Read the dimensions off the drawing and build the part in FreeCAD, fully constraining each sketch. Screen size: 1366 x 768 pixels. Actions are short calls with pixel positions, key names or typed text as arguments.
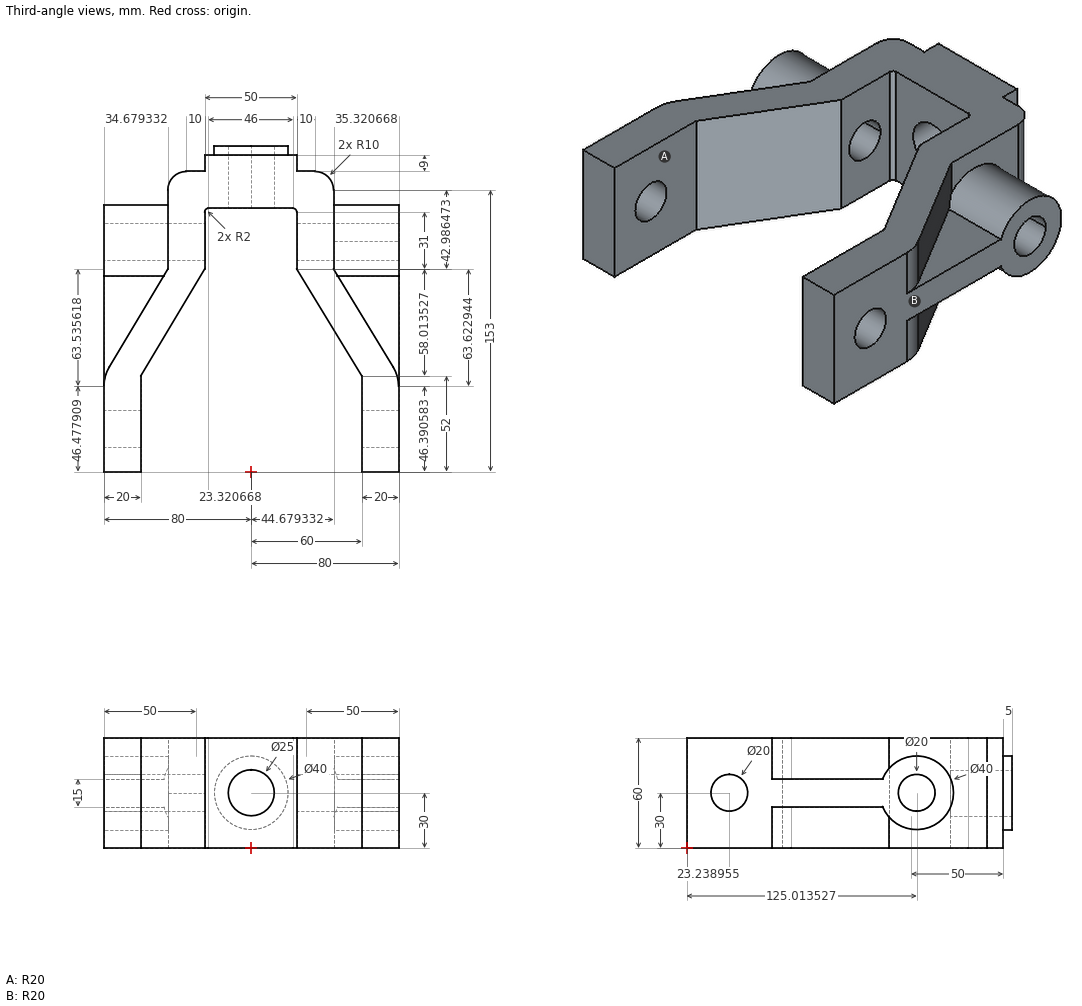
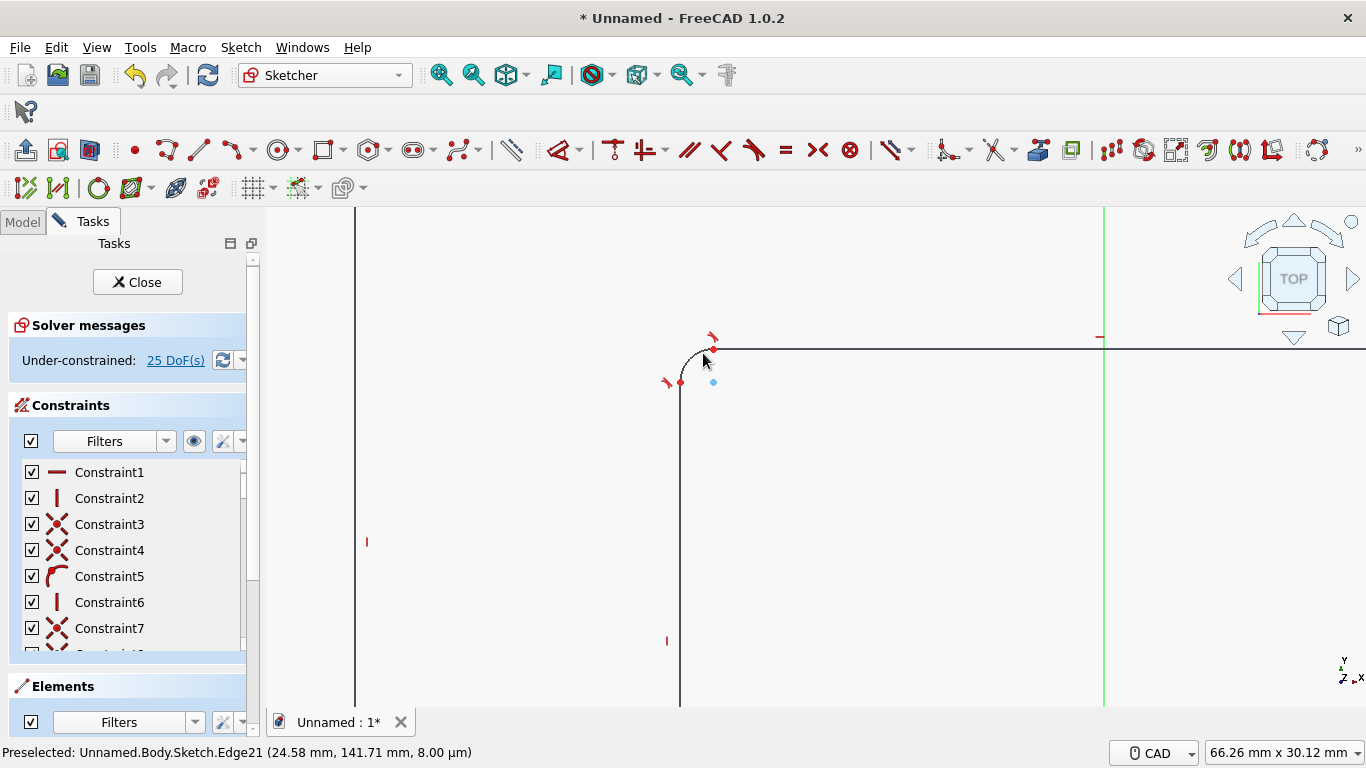
click(699, 353)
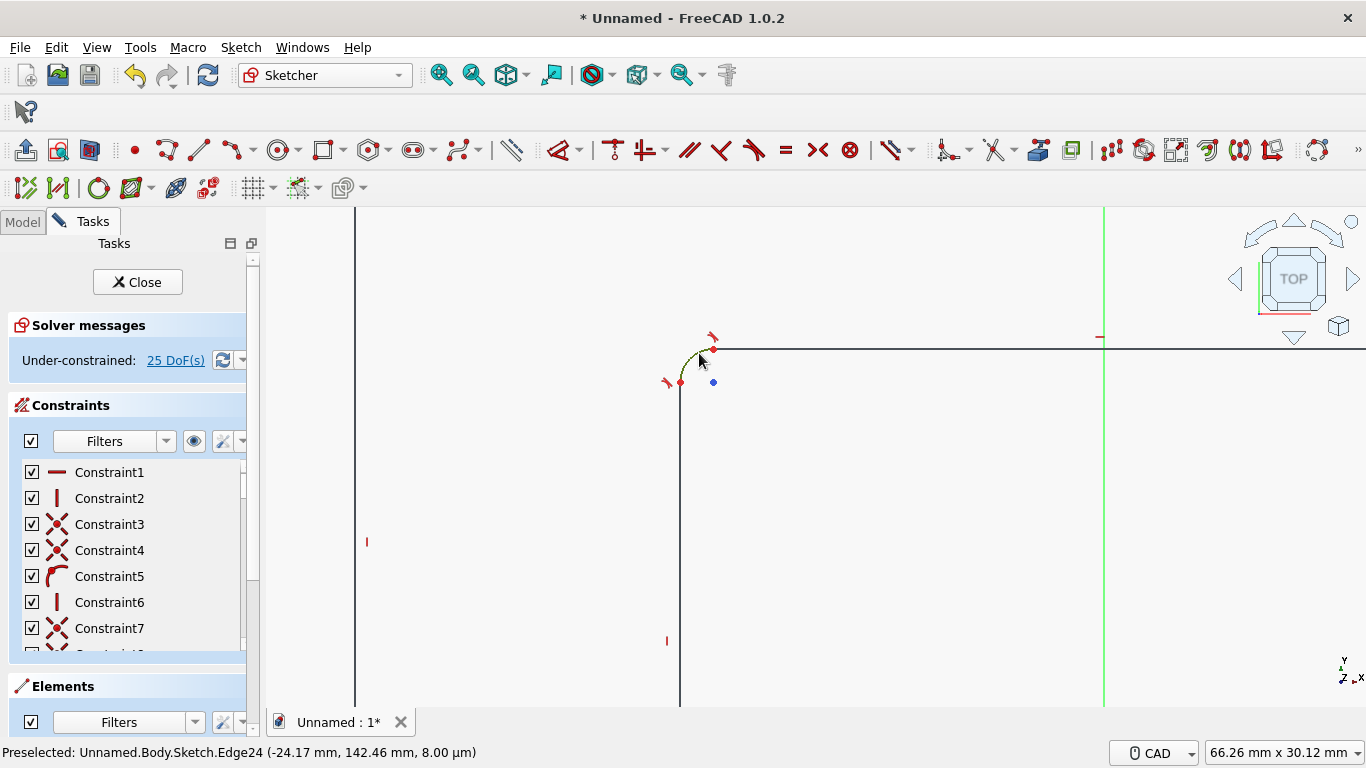
click(786, 150)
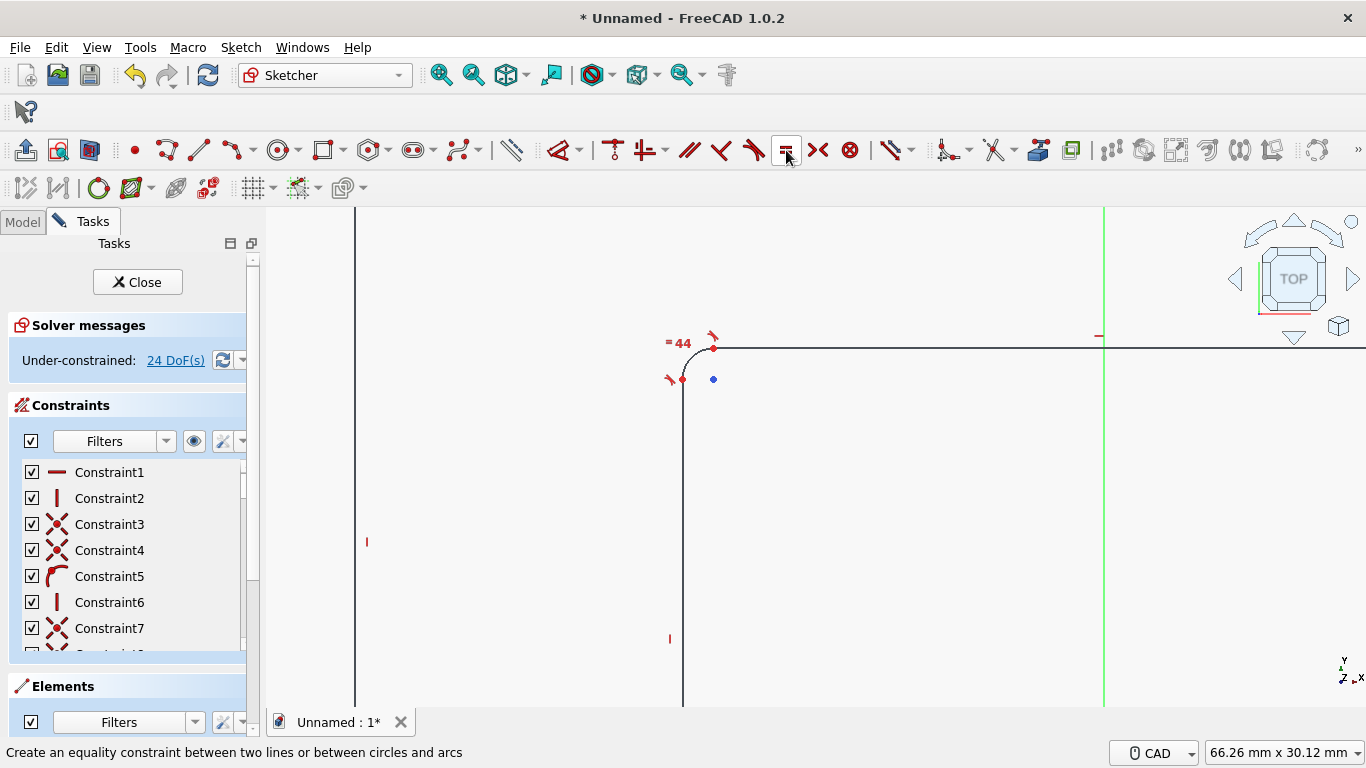
scroll(703, 353, down, 11)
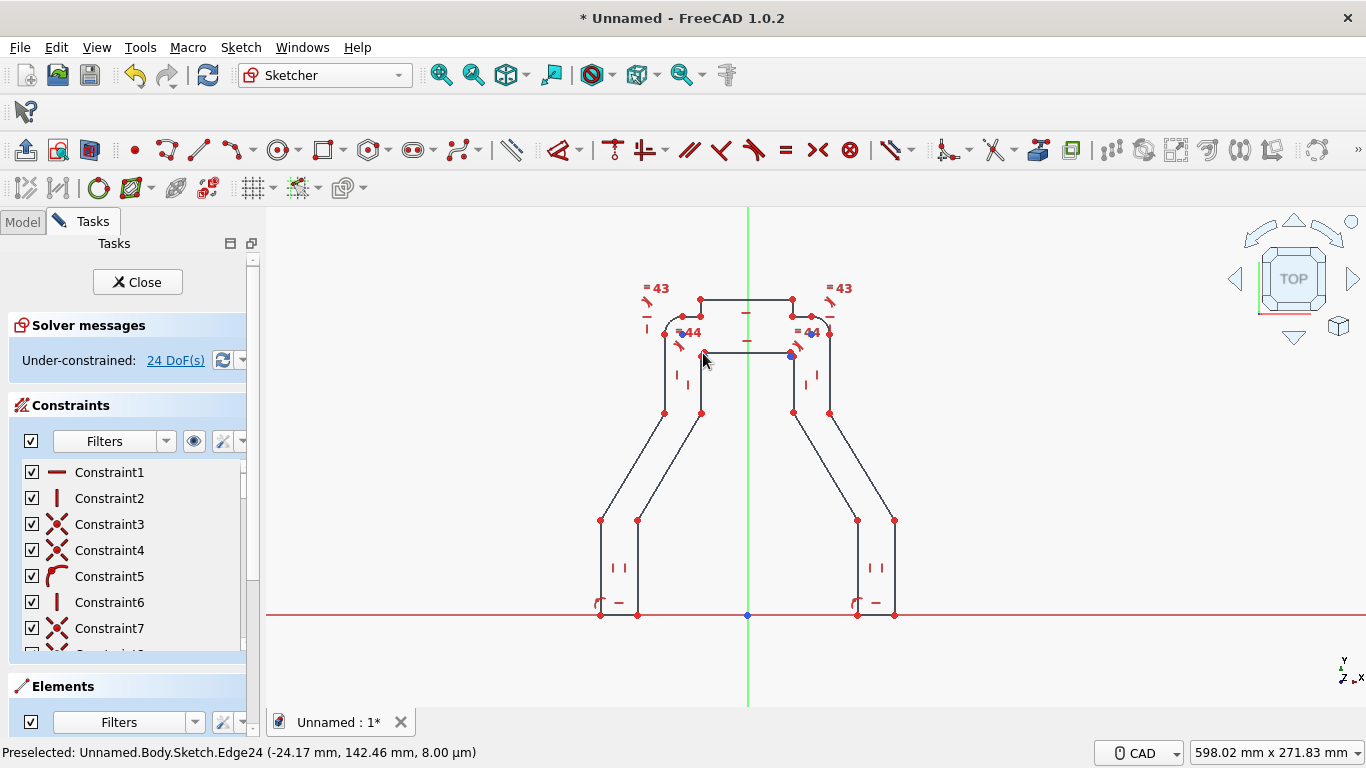
scroll(793, 355, up, 12)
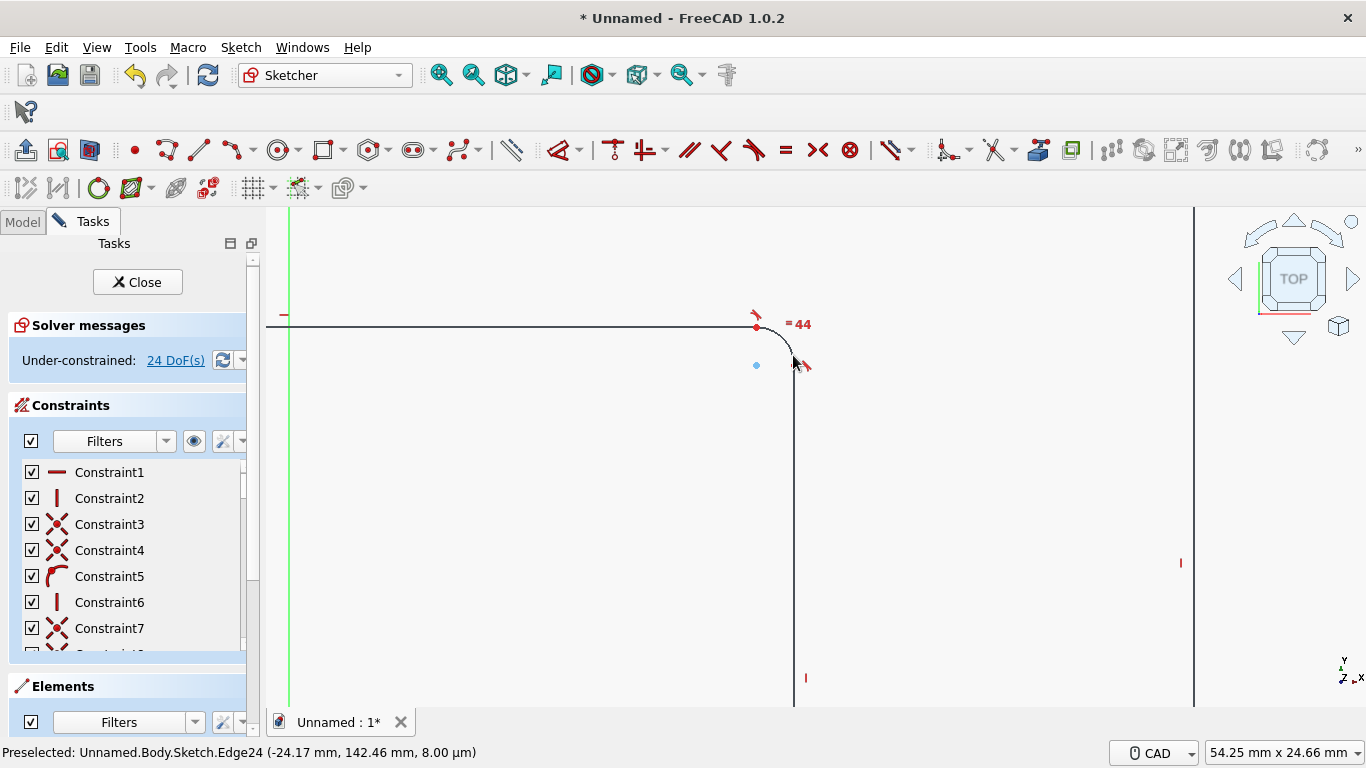
click(790, 348)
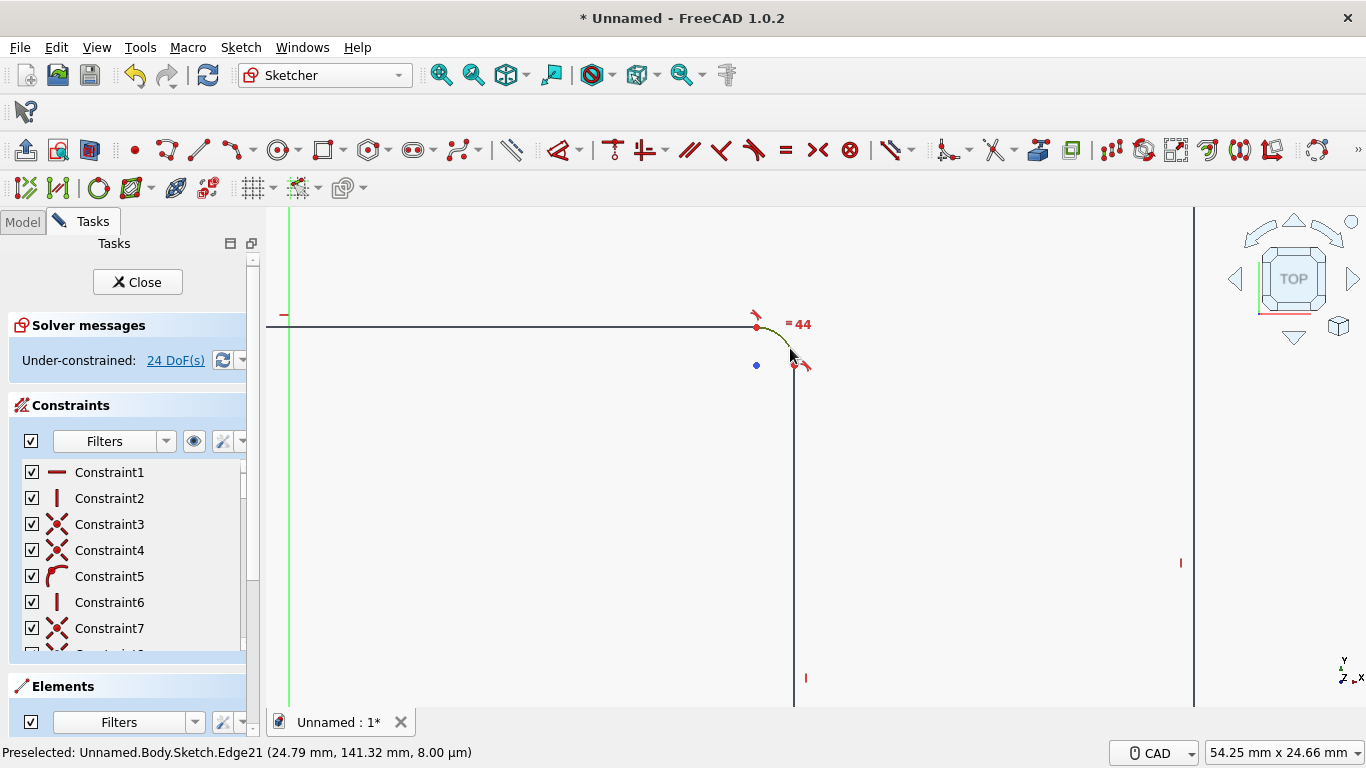
key(k)
key(r)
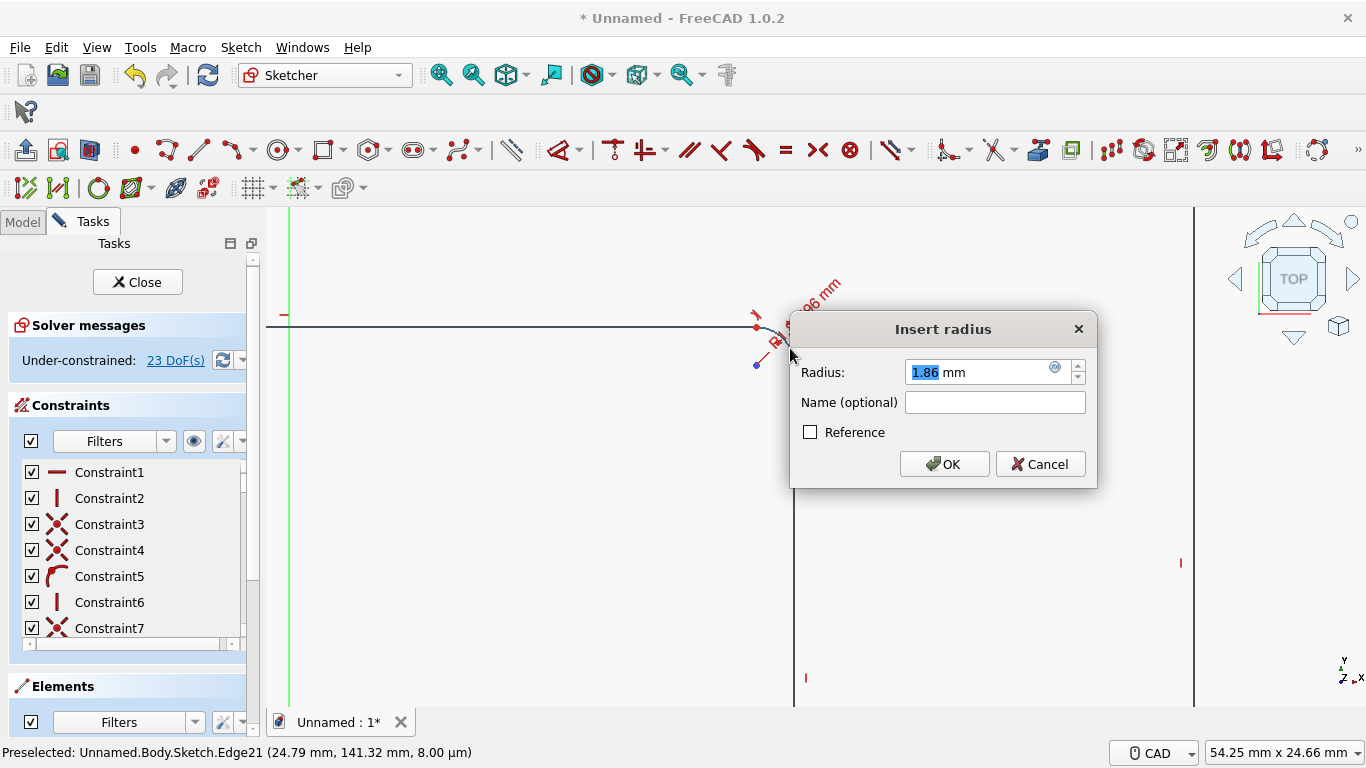
text(2)
key(Return)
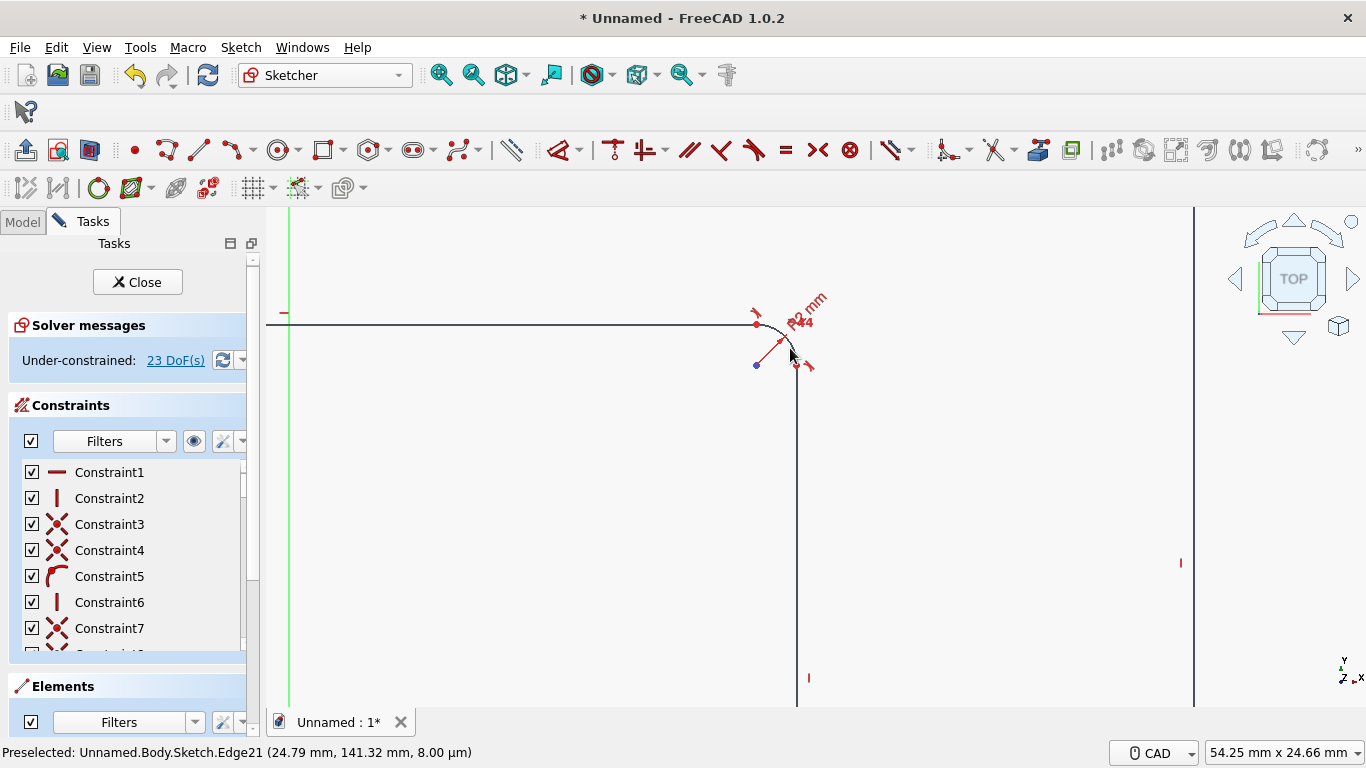
scroll(793, 355, down, 12)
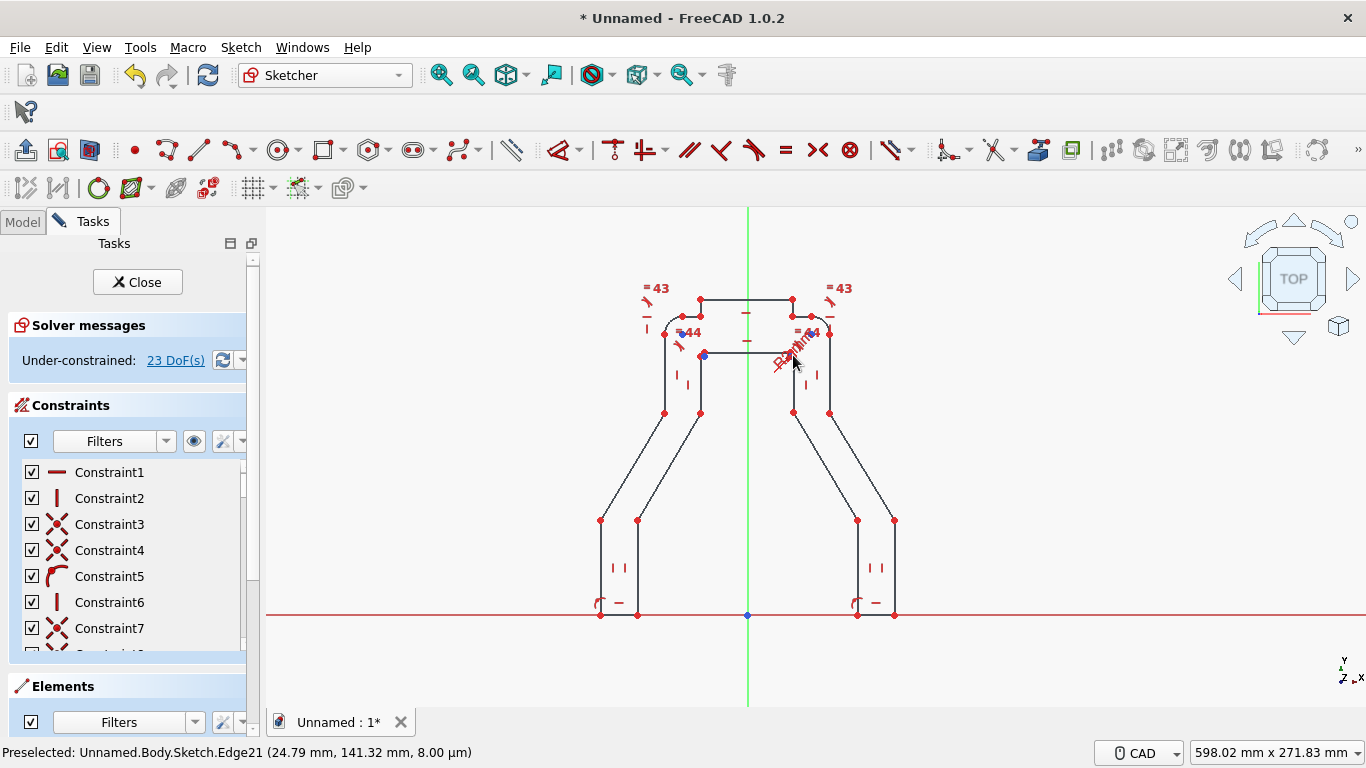
scroll(828, 326, up, 4)